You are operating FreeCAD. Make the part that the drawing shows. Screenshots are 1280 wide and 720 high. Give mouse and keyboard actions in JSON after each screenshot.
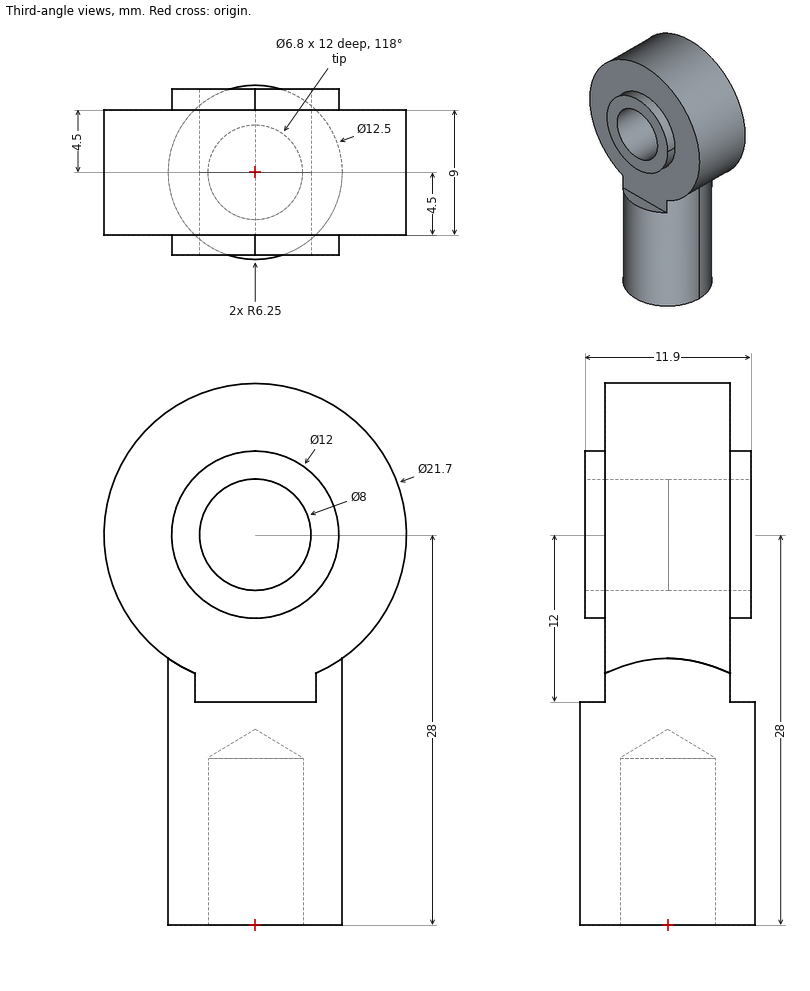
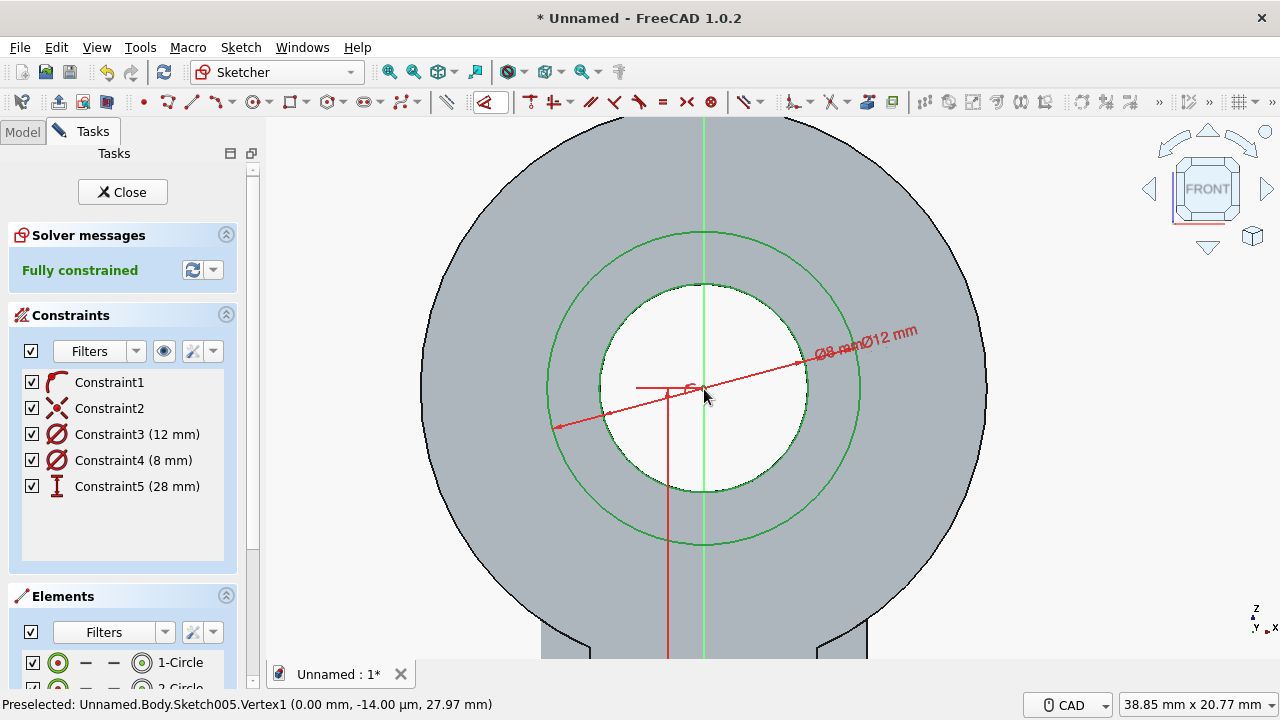
{"action": "left_click", "coordinate": [123, 192]}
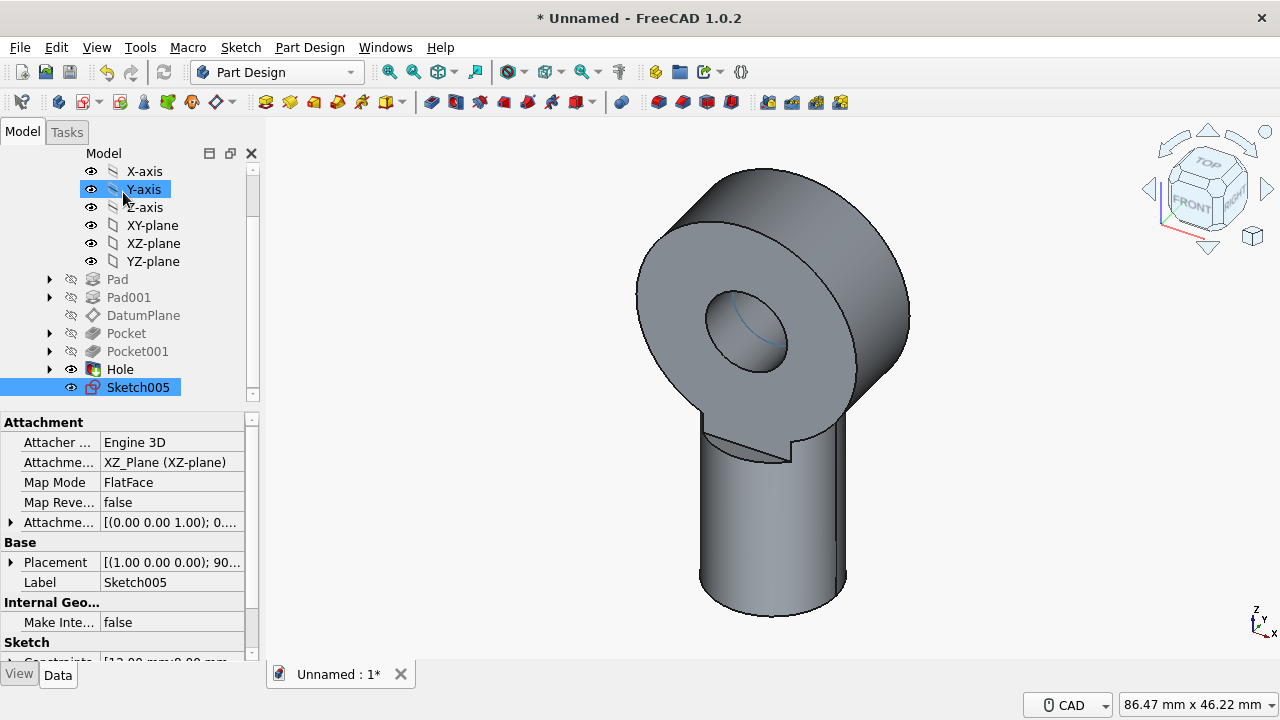
{"action": "left_click", "coordinate": [266, 102]}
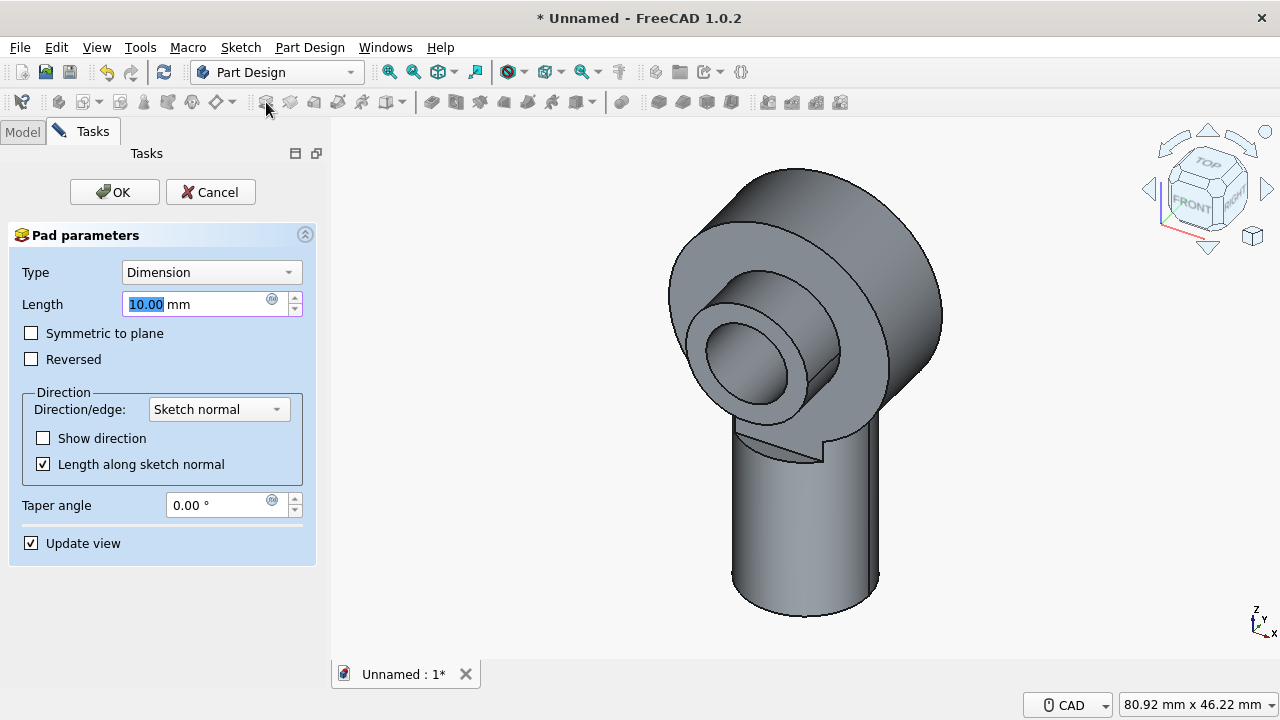
{"action": "type", "text": "11.9"}
{"action": "key", "text": "Tab"}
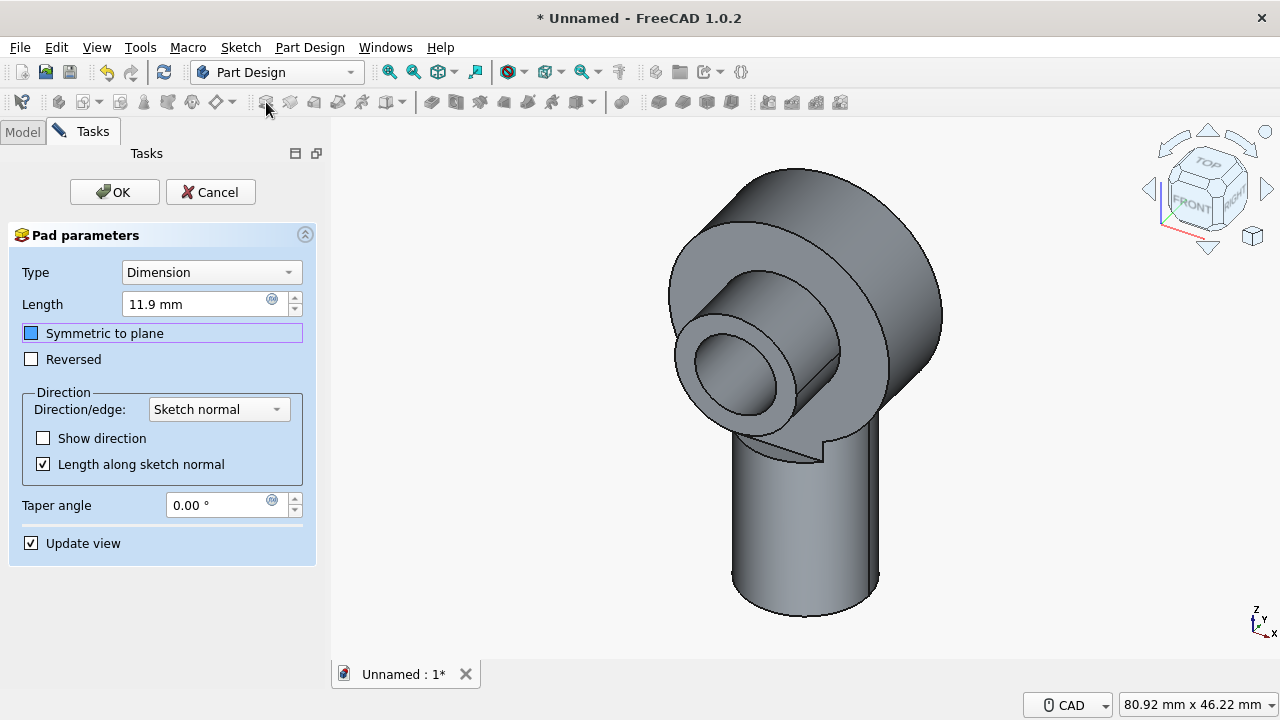
{"action": "left_click", "coordinate": [30, 333]}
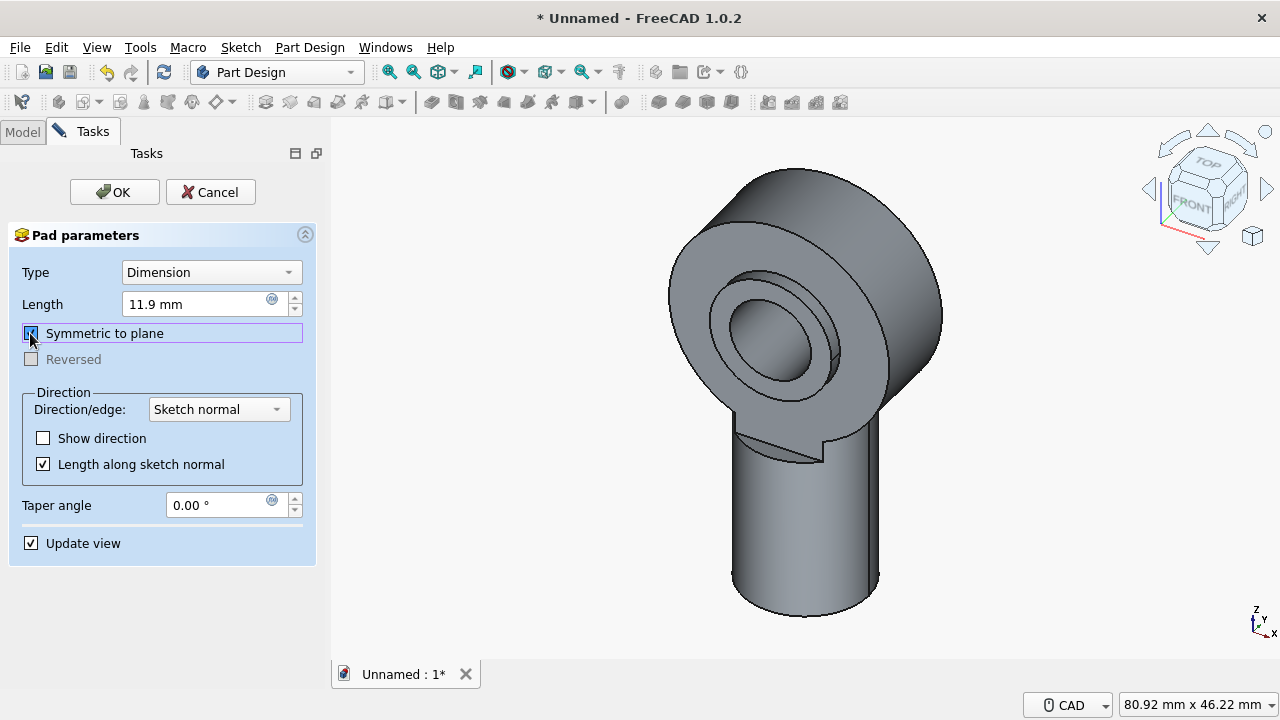
{"action": "left_click", "coordinate": [115, 192]}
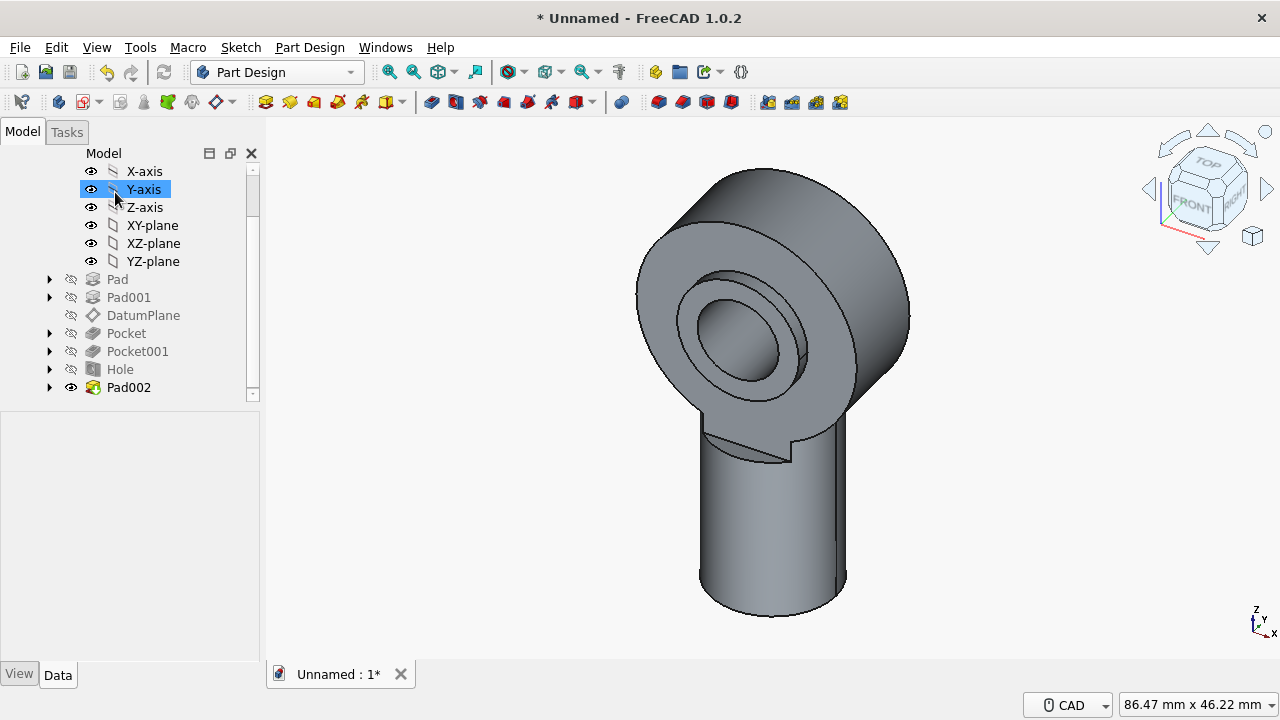
{"action": "key", "text": "0"}